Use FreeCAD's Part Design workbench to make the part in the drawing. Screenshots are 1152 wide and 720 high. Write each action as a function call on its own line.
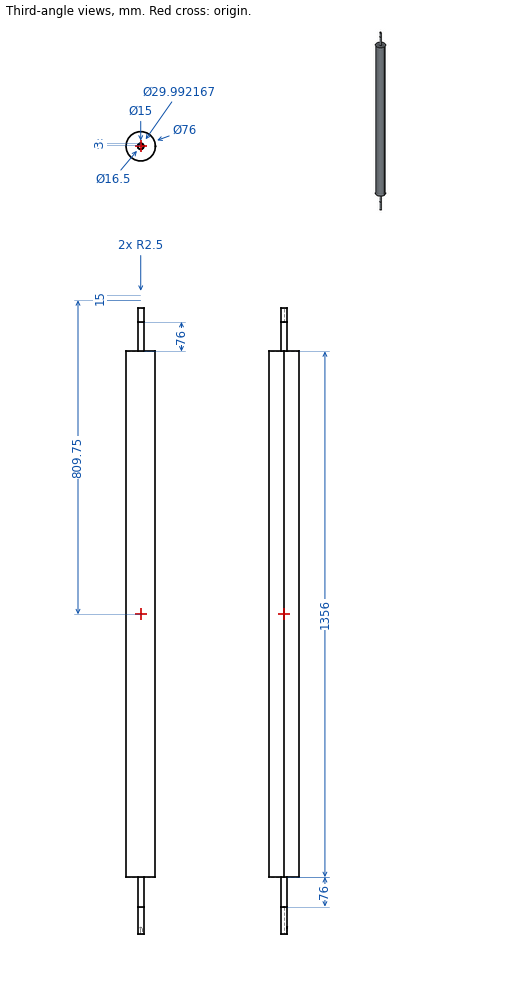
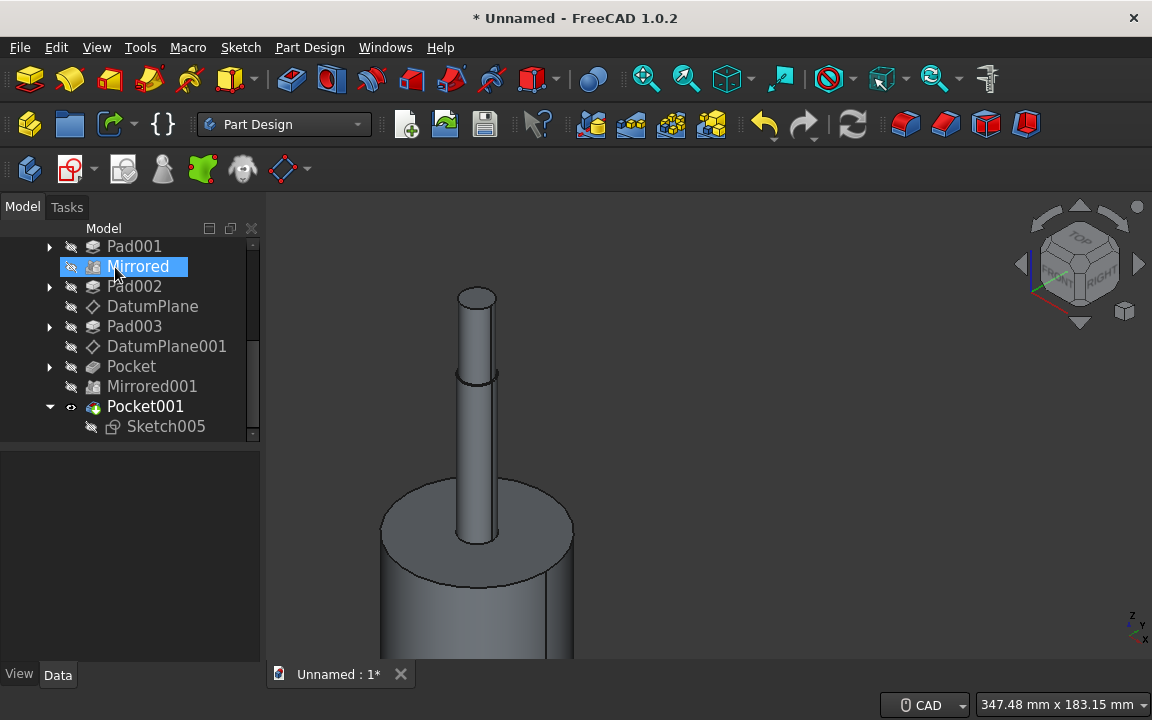
click(648, 80)